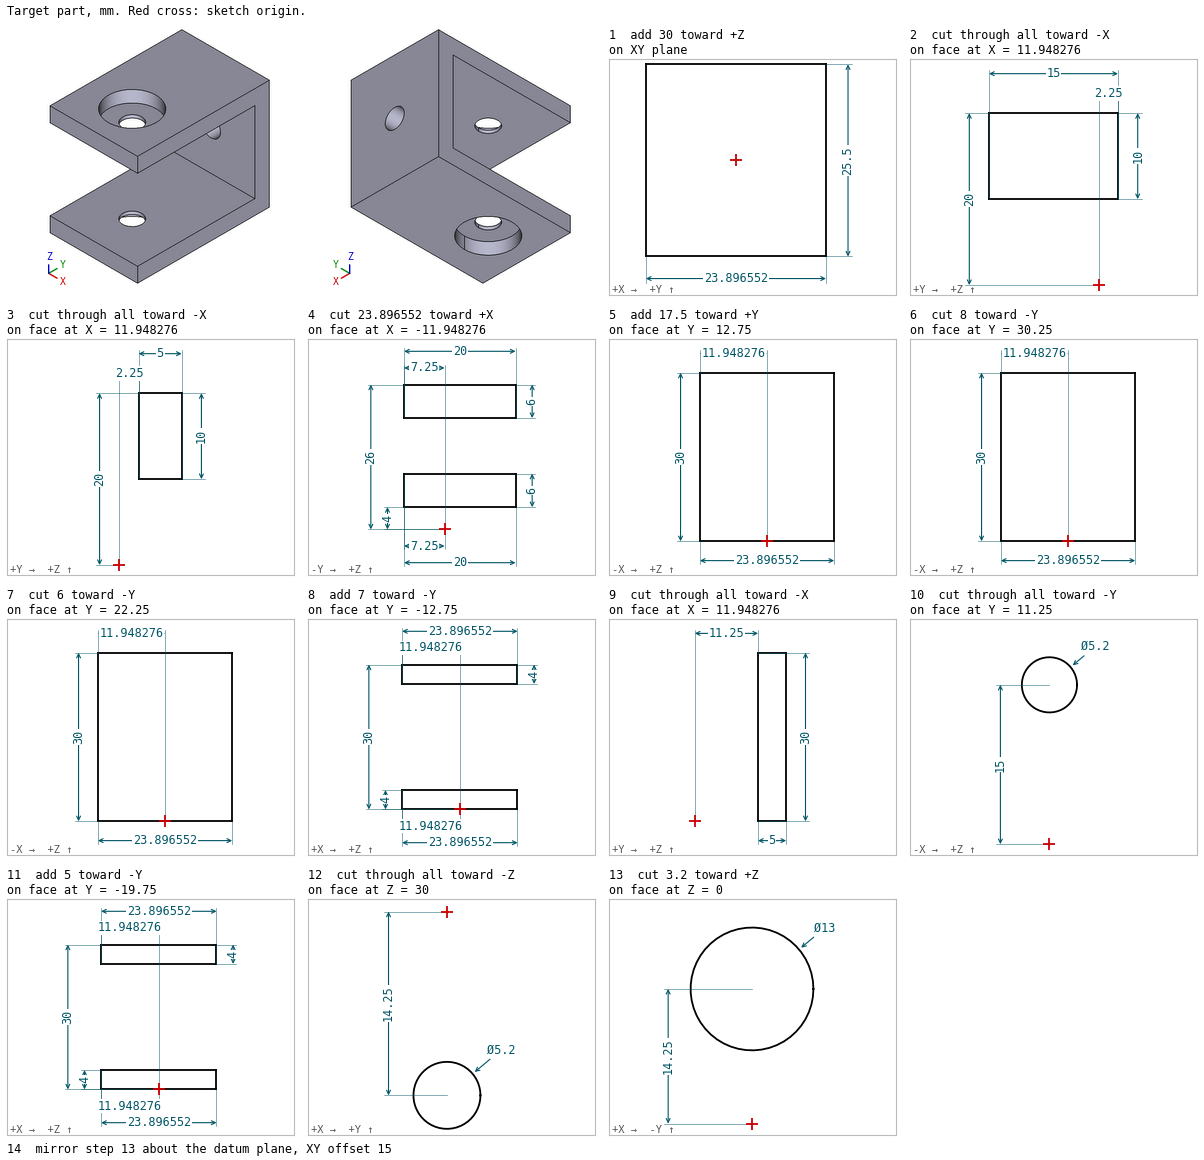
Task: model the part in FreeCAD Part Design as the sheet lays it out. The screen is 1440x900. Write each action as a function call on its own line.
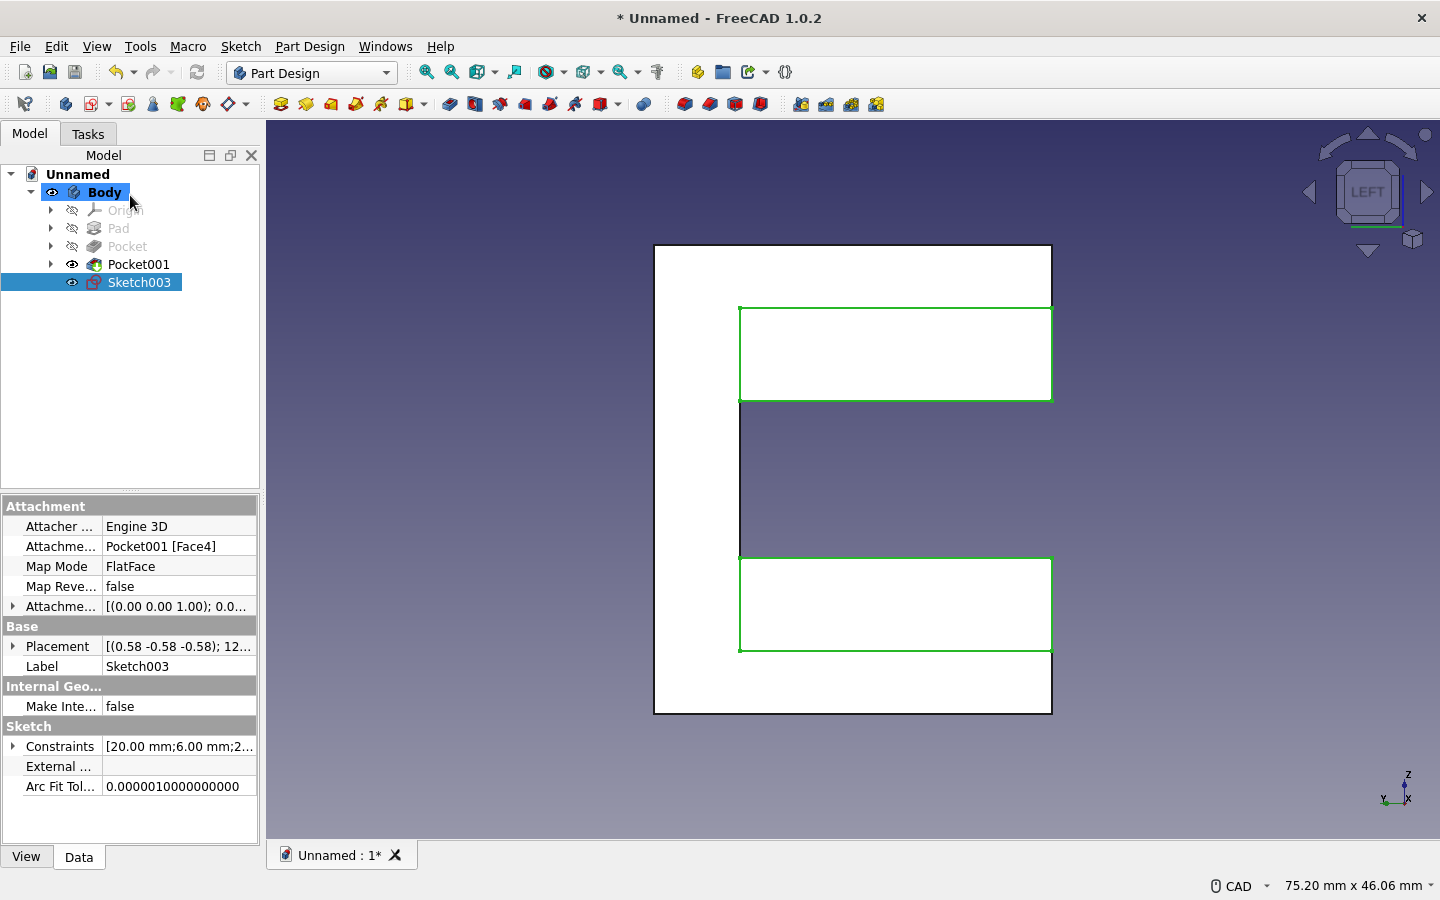
click(450, 104)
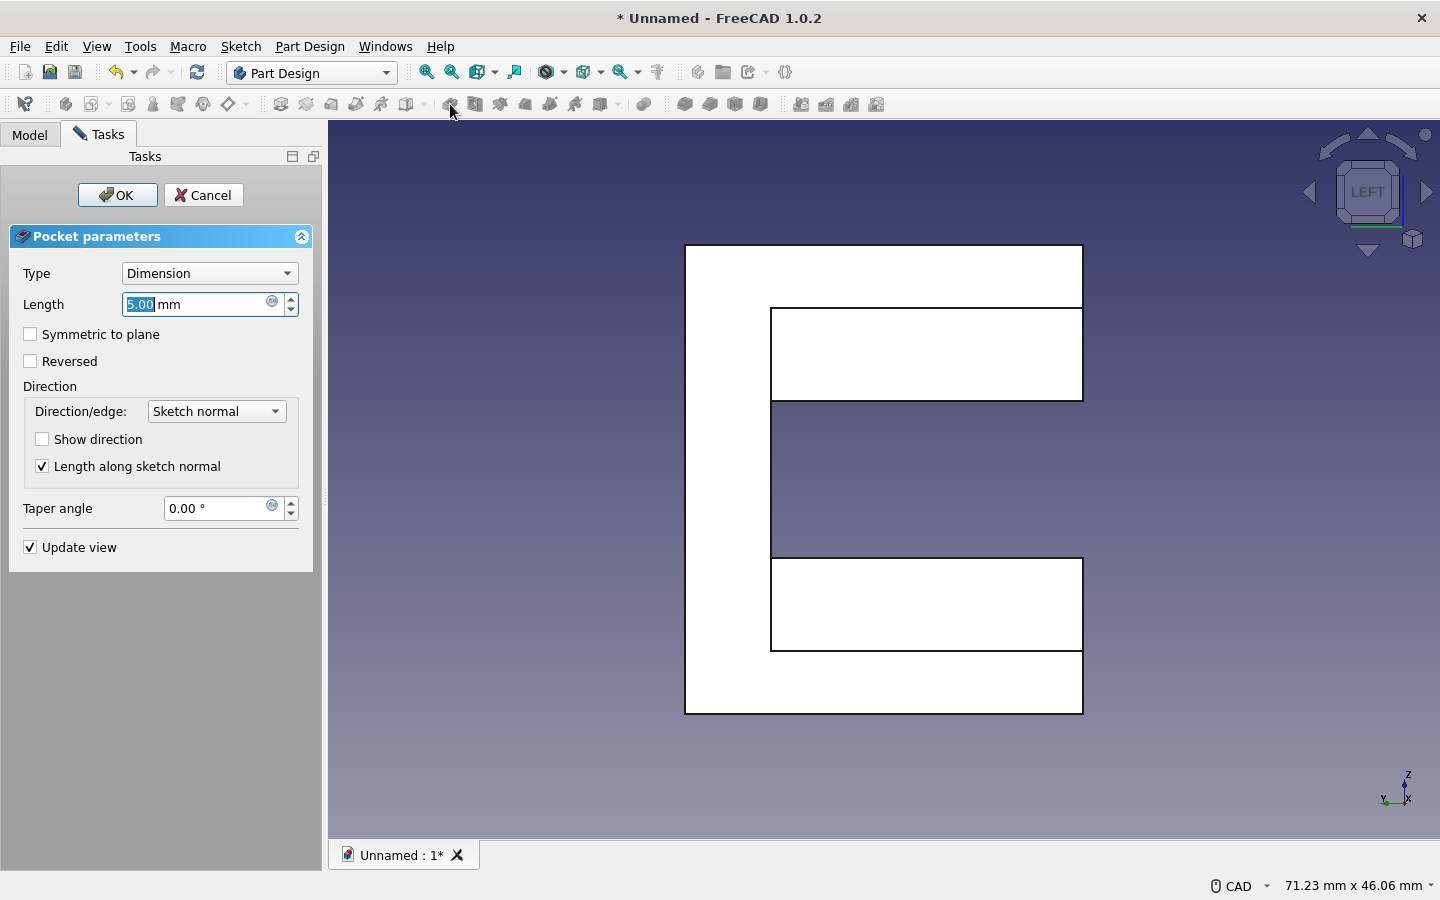
text(23.896552)
key(Tab)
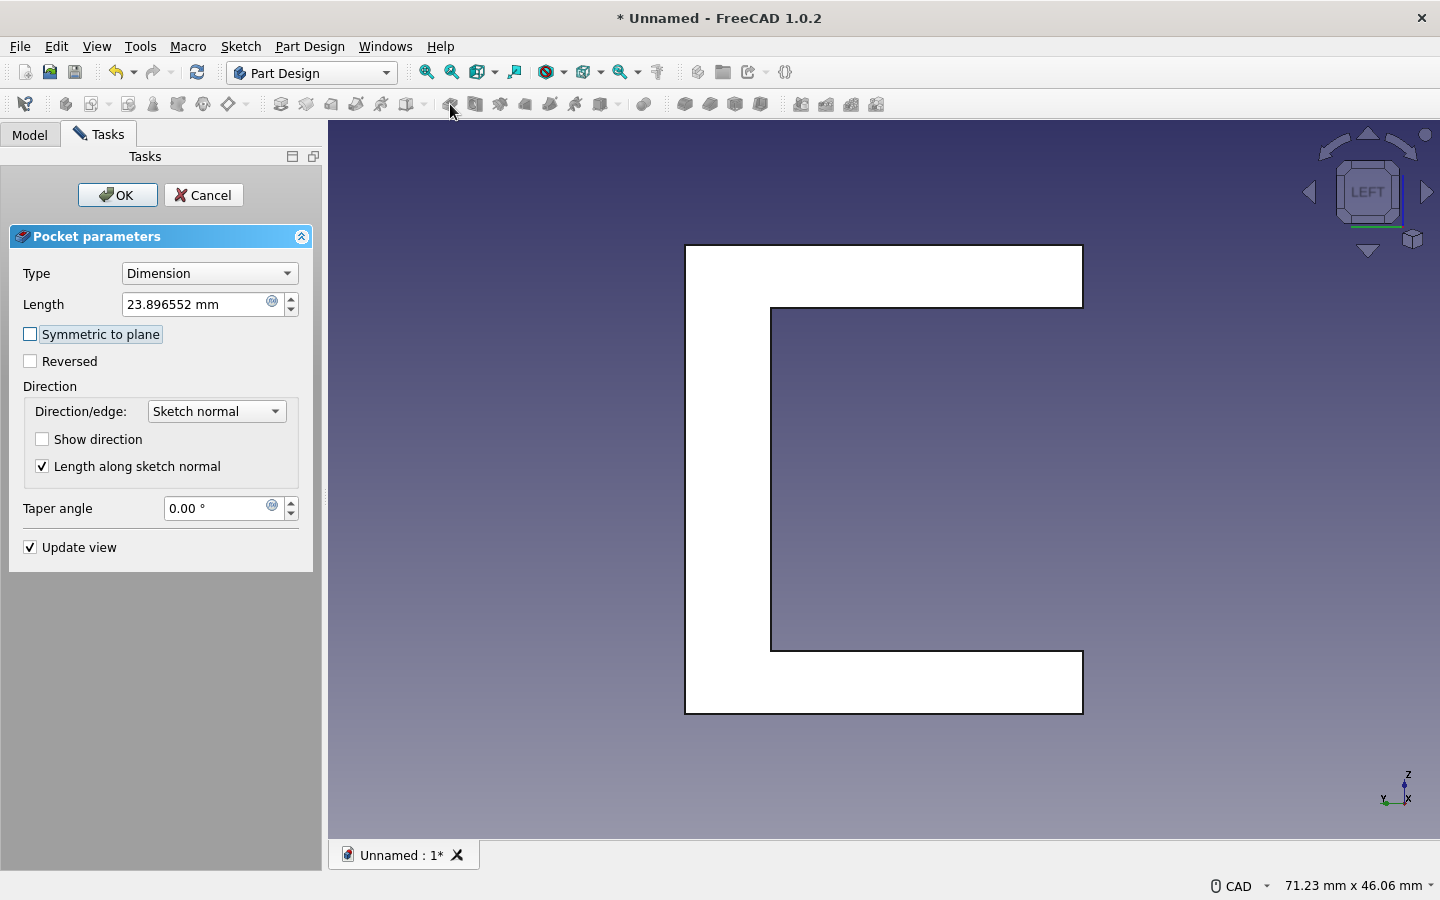
click(118, 195)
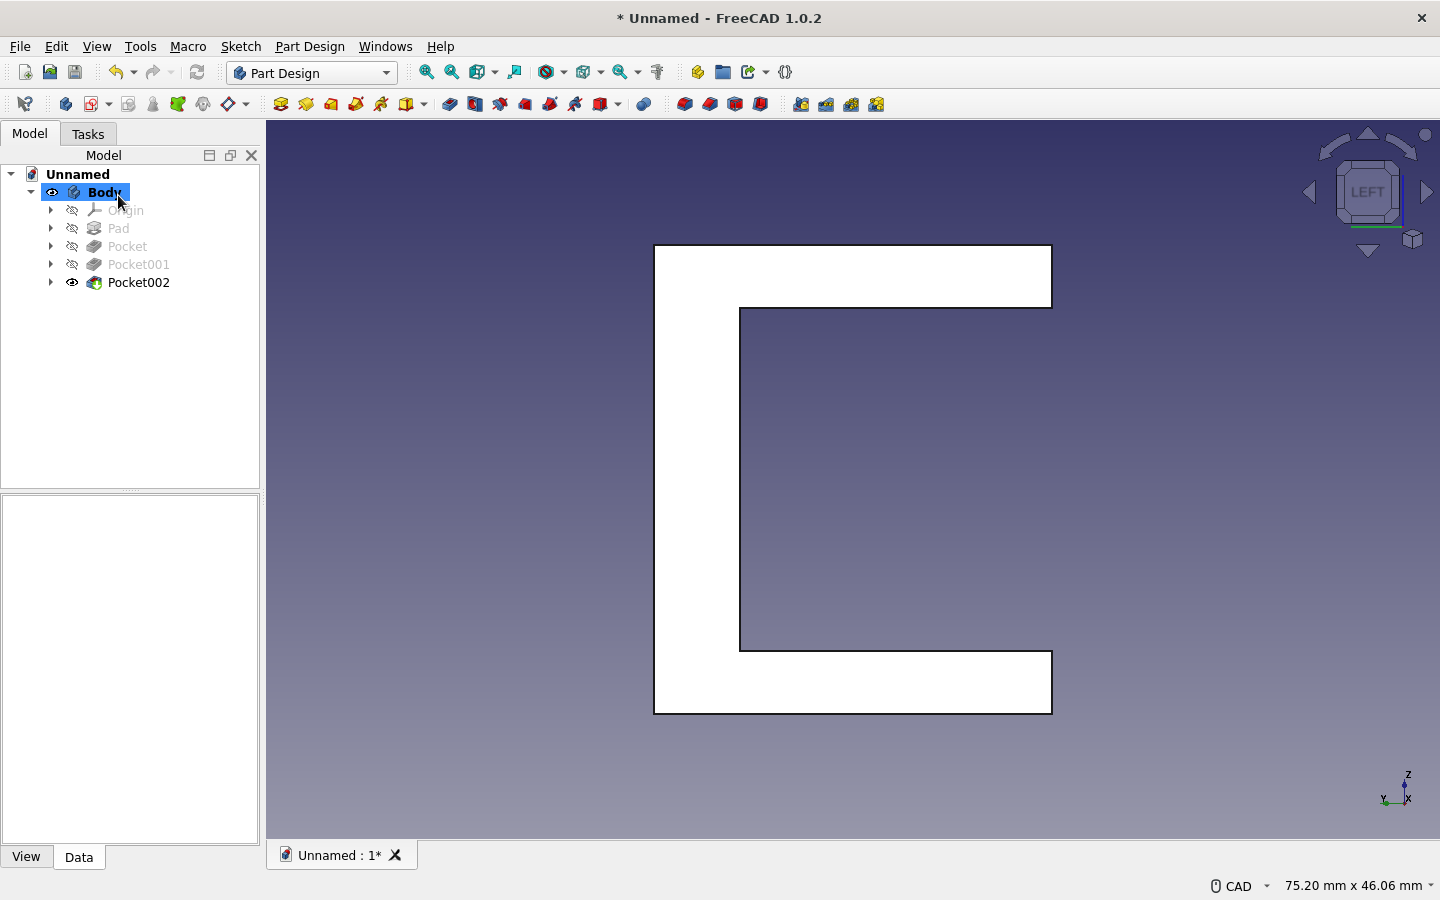
key(4)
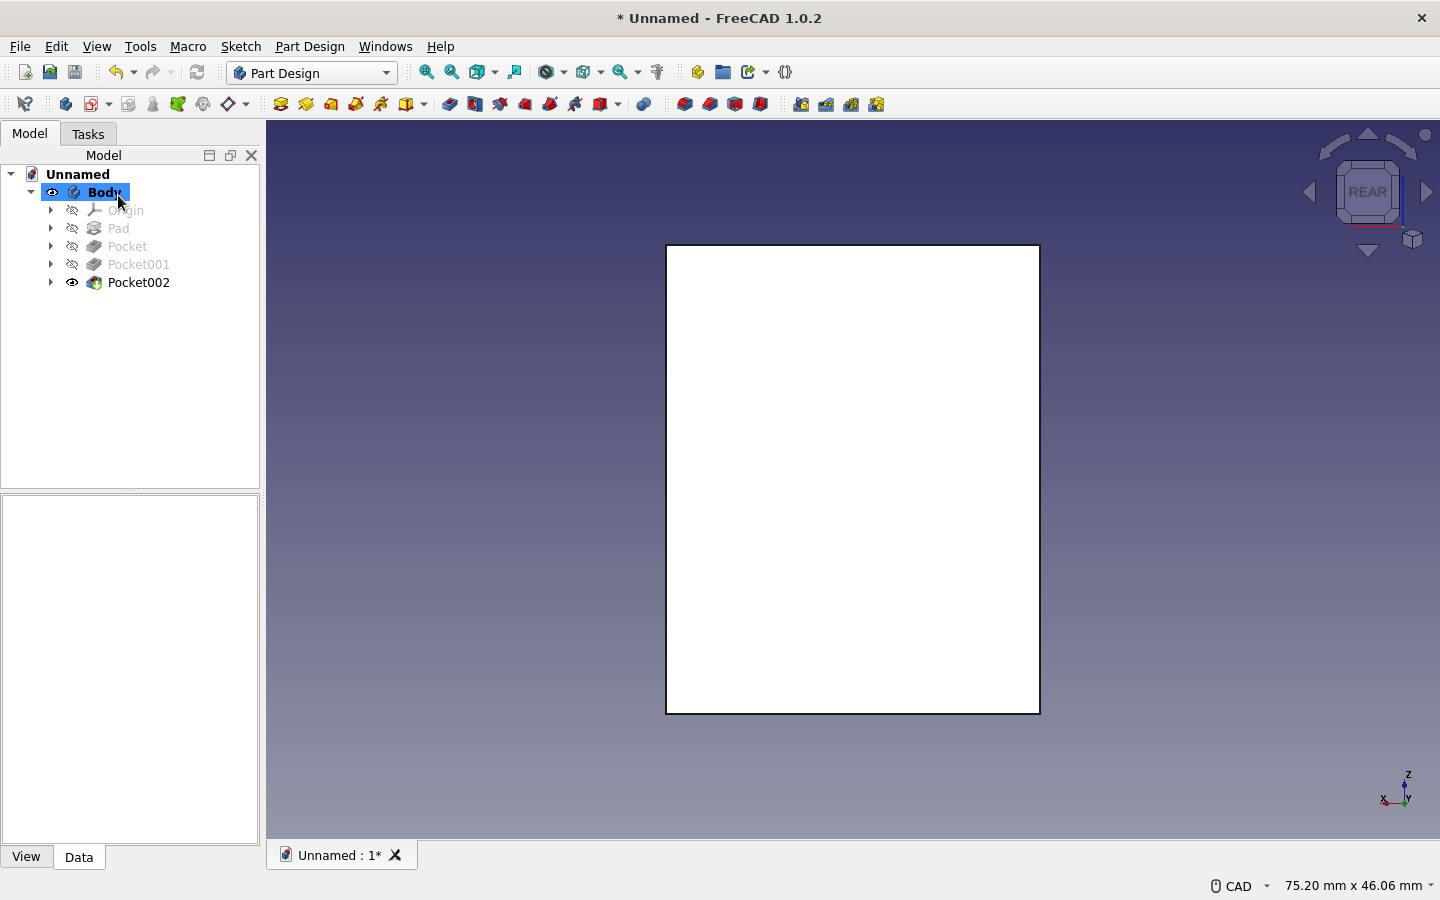
click(853, 479)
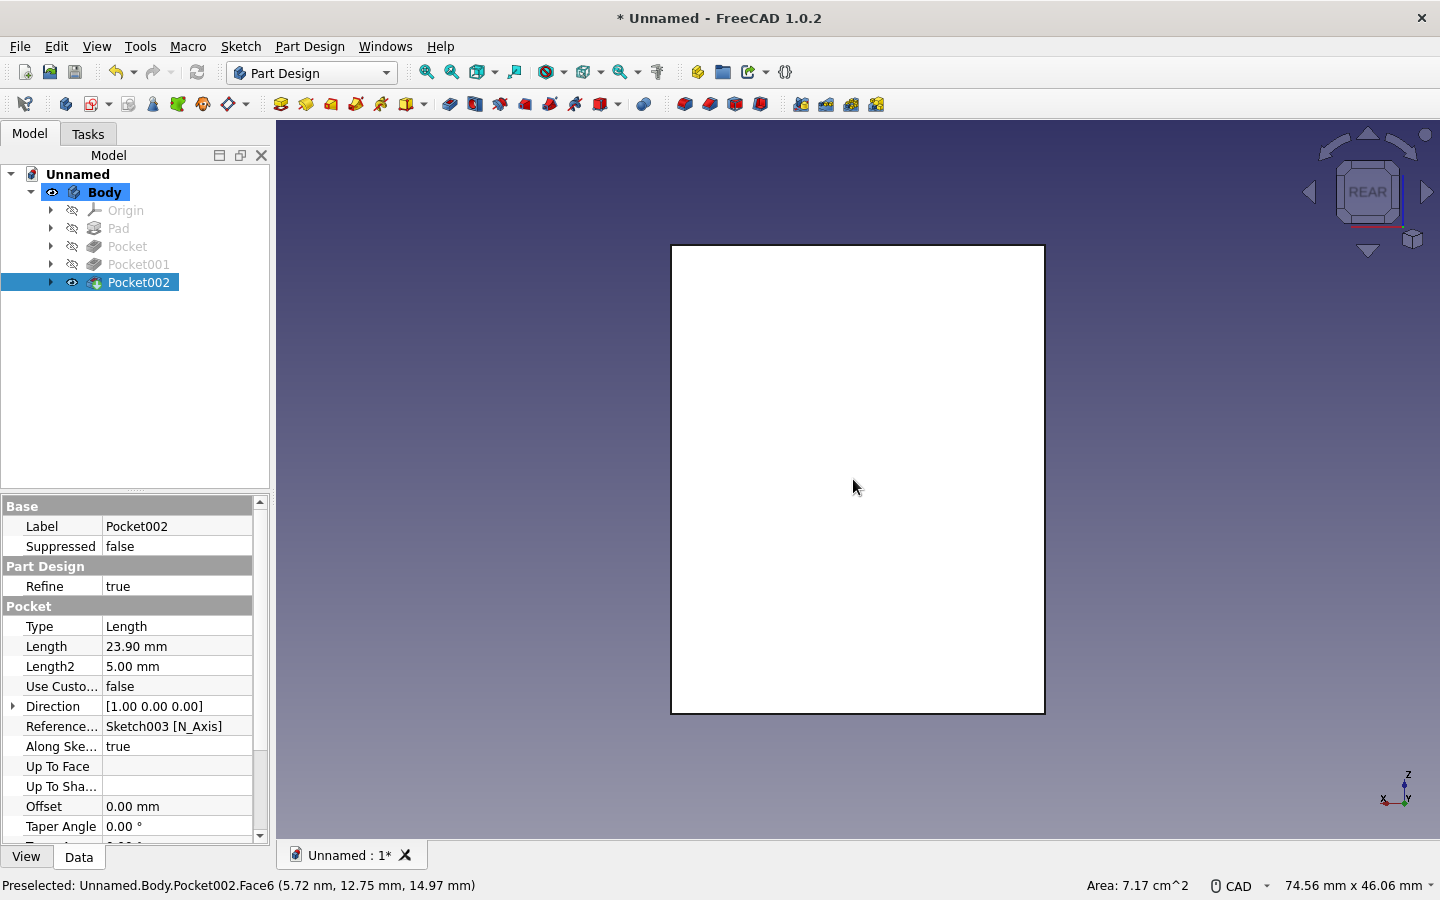
click(90, 104)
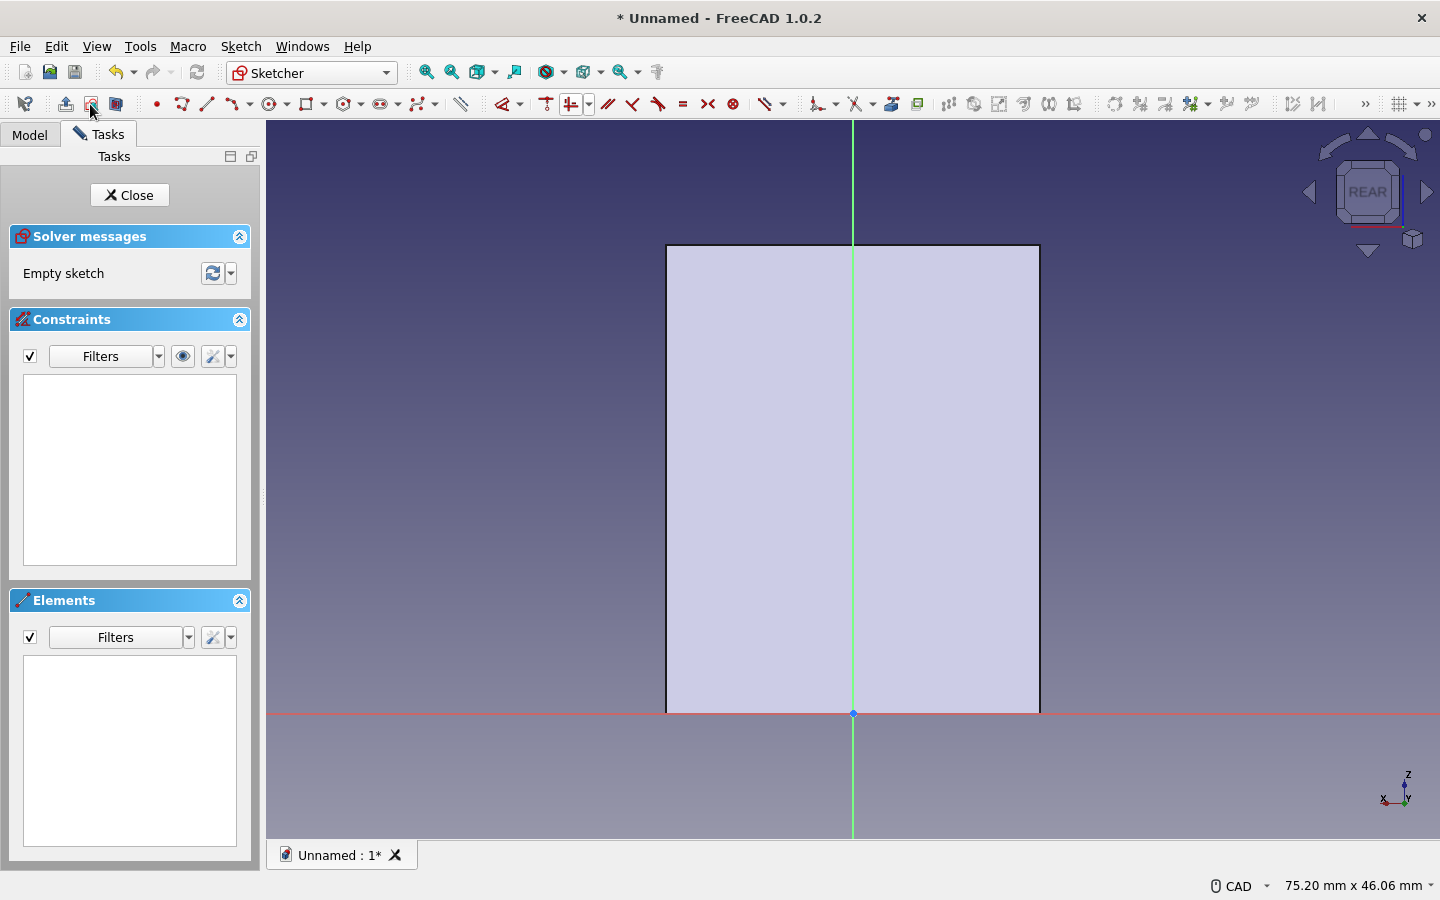
key(g)
key(r)